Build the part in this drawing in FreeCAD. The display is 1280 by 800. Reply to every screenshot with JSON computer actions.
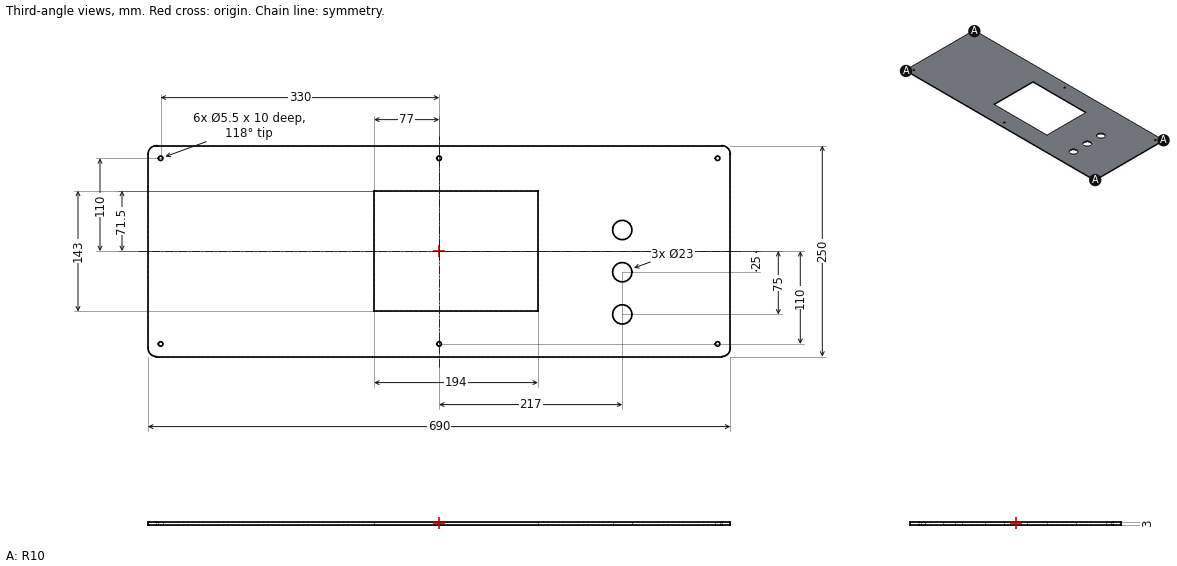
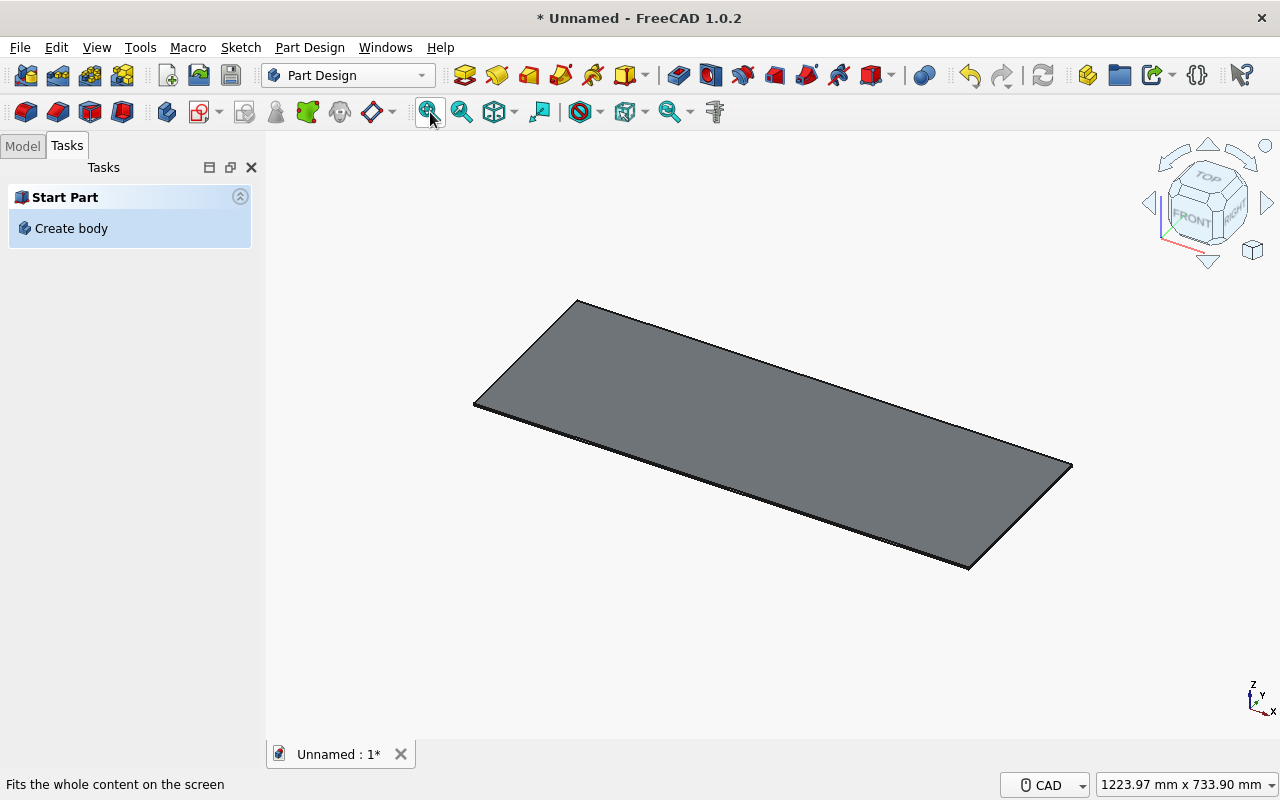
{"action": "left_click", "coordinate": [914, 480]}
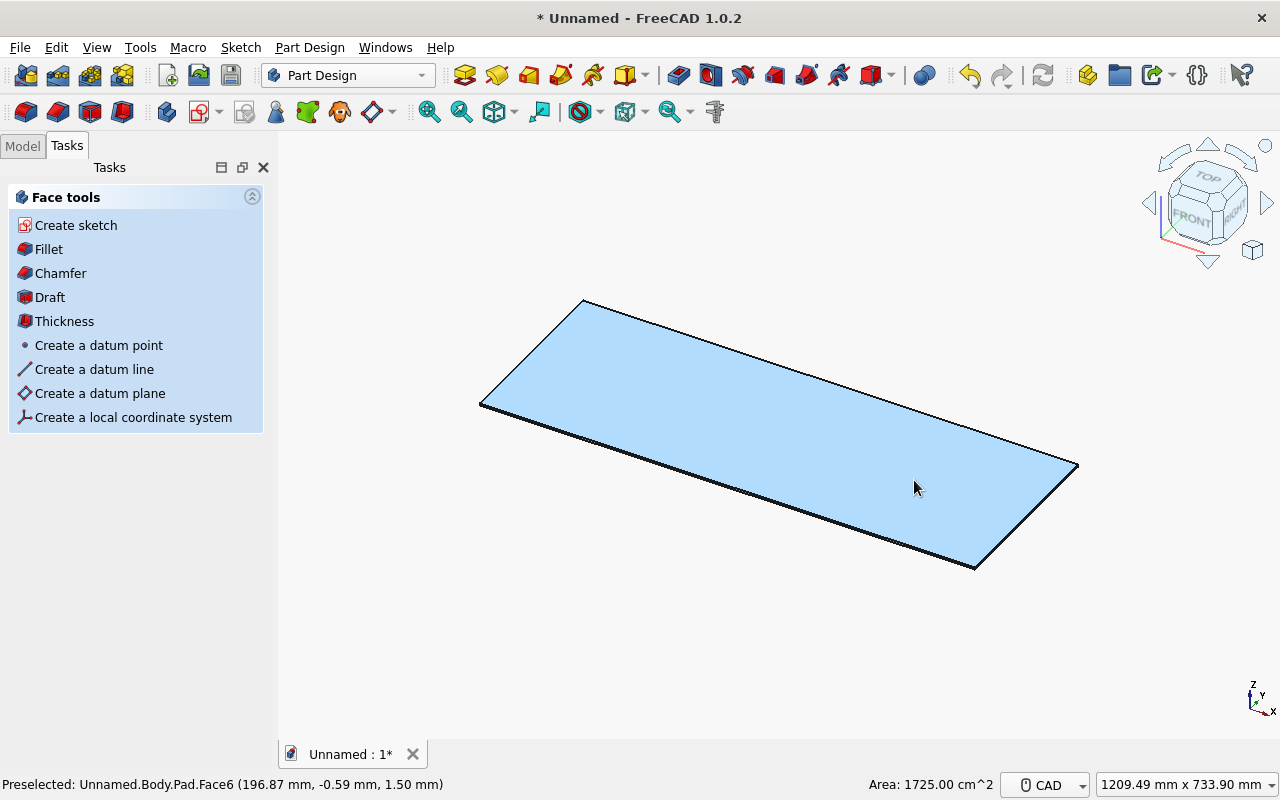
{"action": "left_click", "coordinate": [200, 112]}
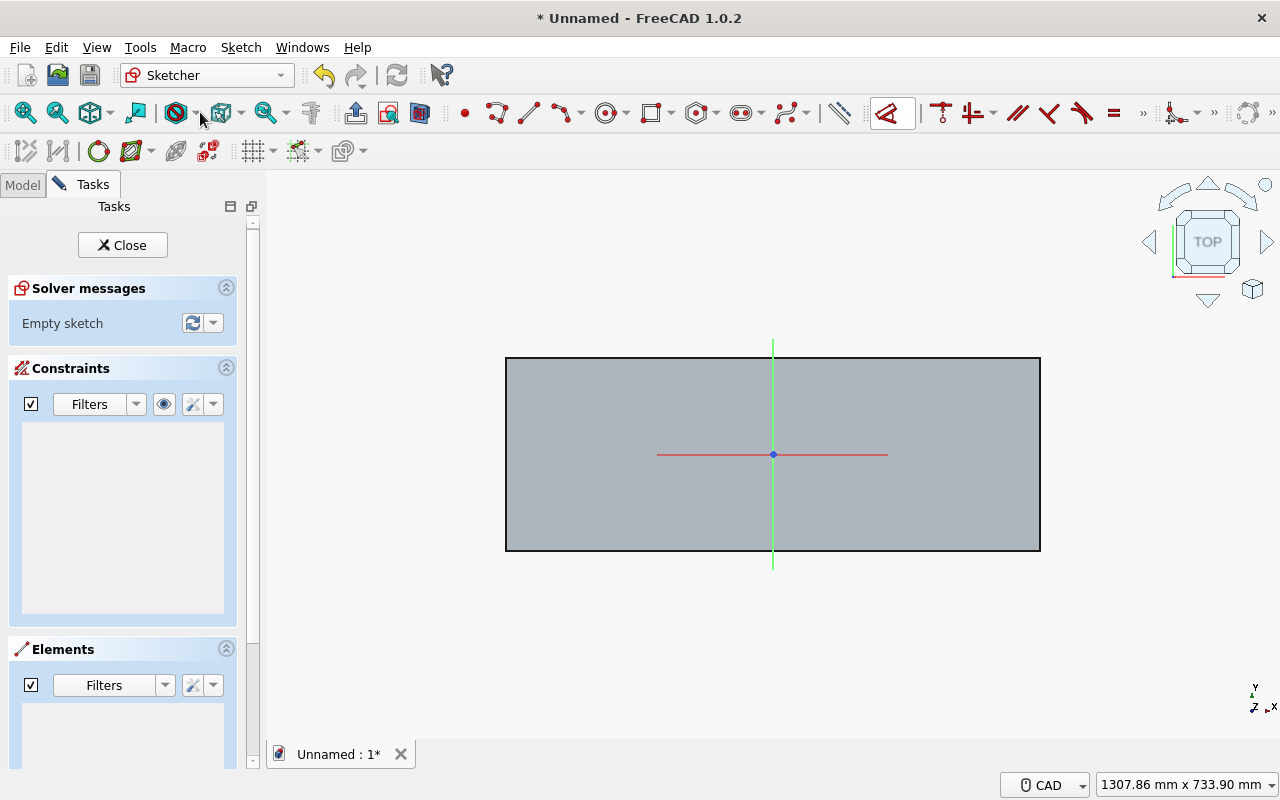
{"action": "scroll", "coordinate": [825, 455], "scroll_direction": "up", "scroll_amount": 6}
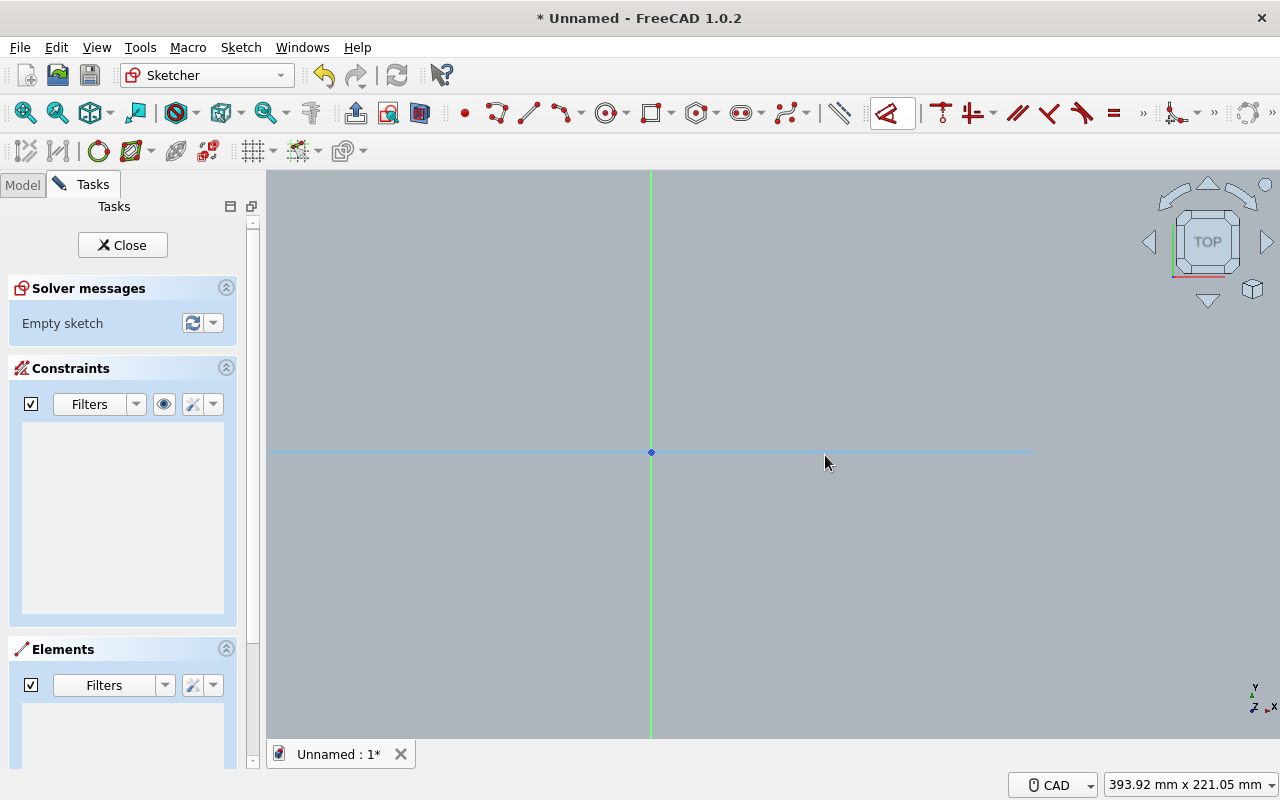
{"action": "left_click", "coordinate": [652, 114]}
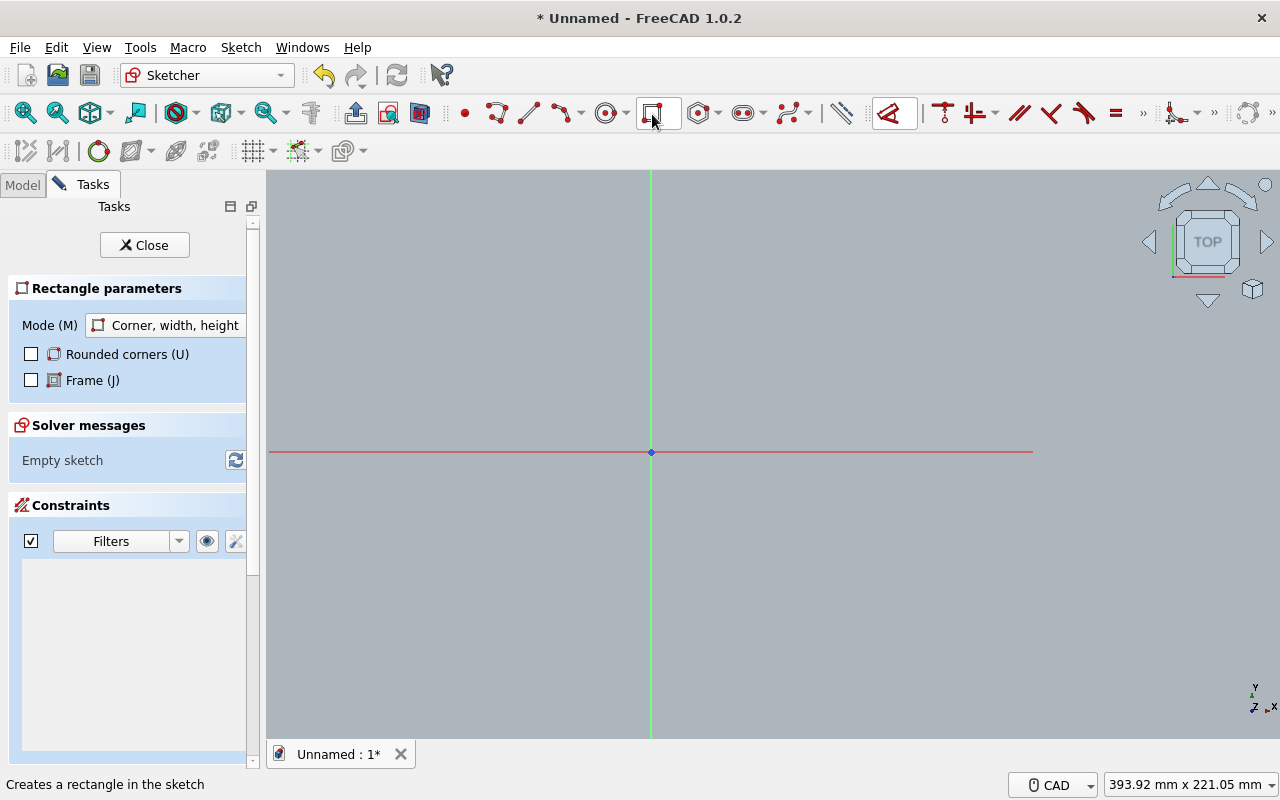
{"action": "left_click", "coordinate": [453, 268]}
{"action": "left_click", "coordinate": [952, 636]}
{"action": "key", "text": "Escape"}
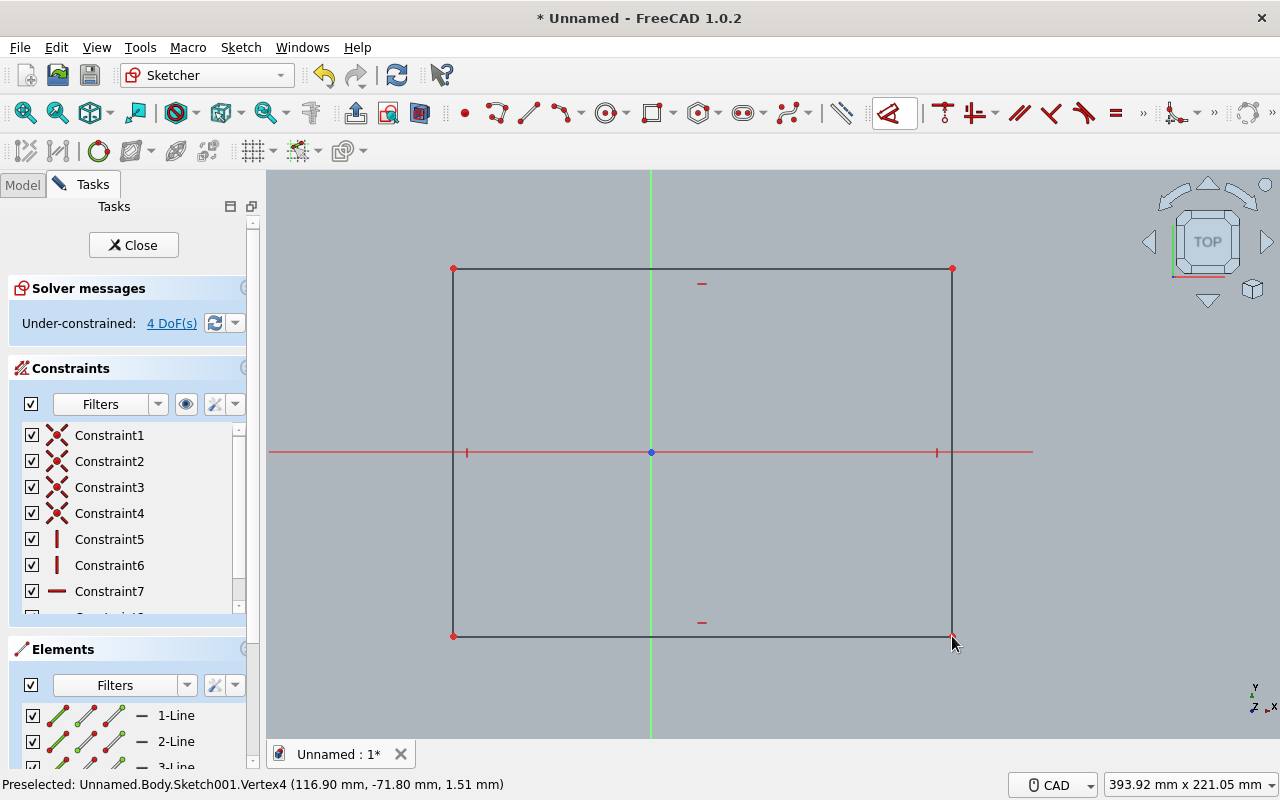
{"action": "left_click", "coordinate": [453, 379]}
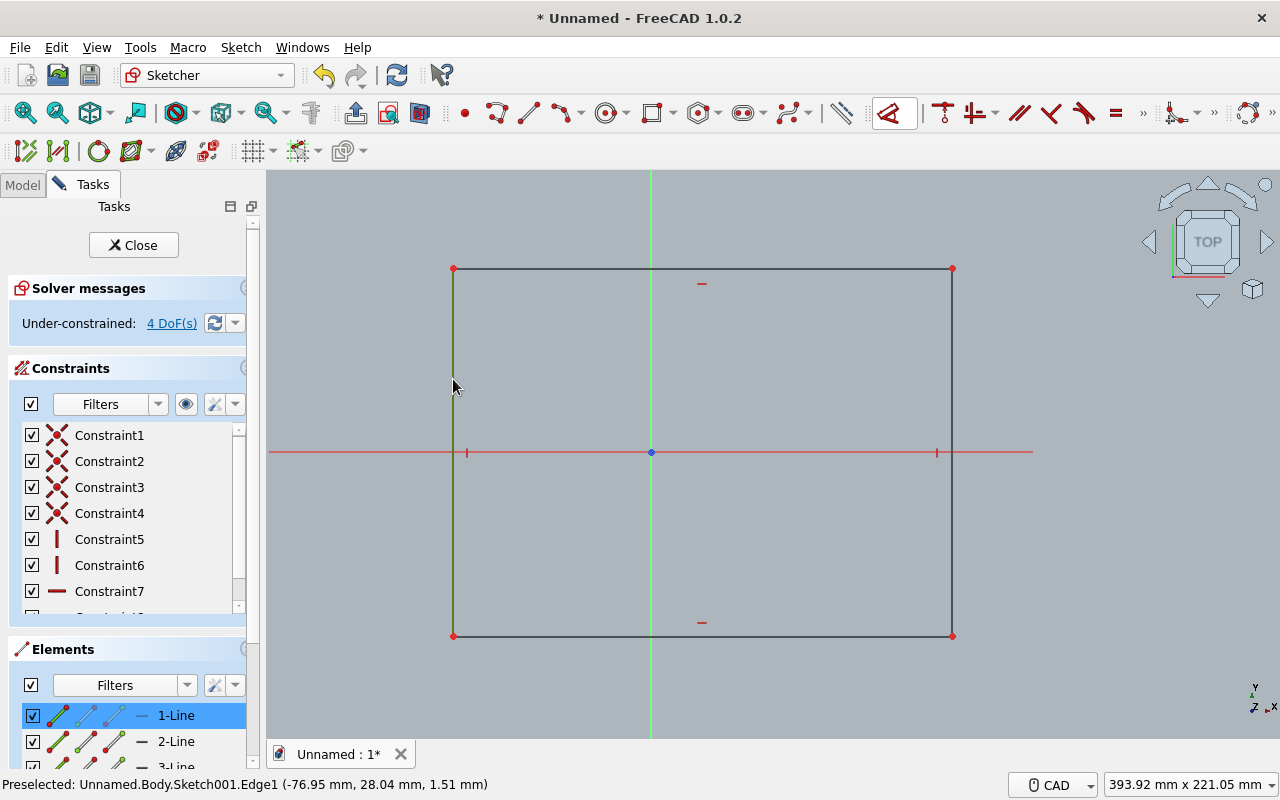
{"action": "left_click", "coordinate": [912, 114]}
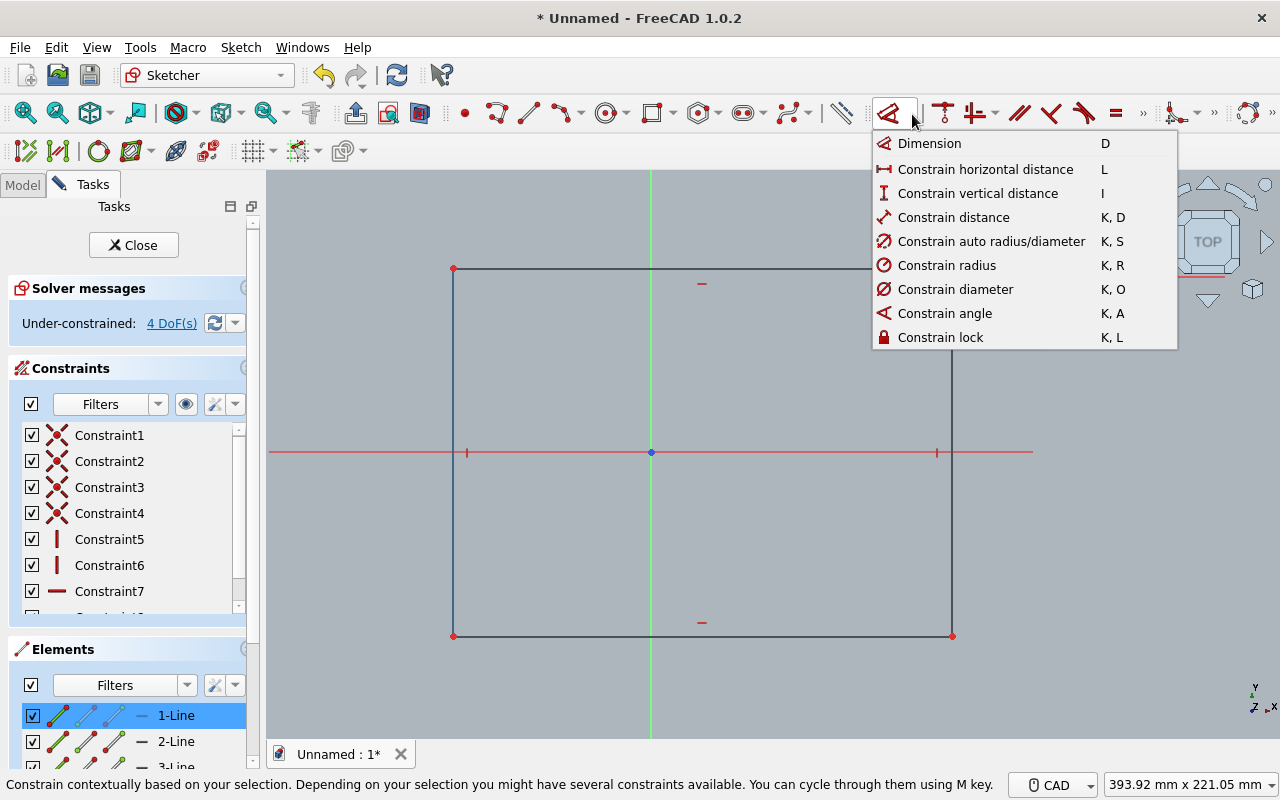
{"action": "left_click", "coordinate": [1025, 193]}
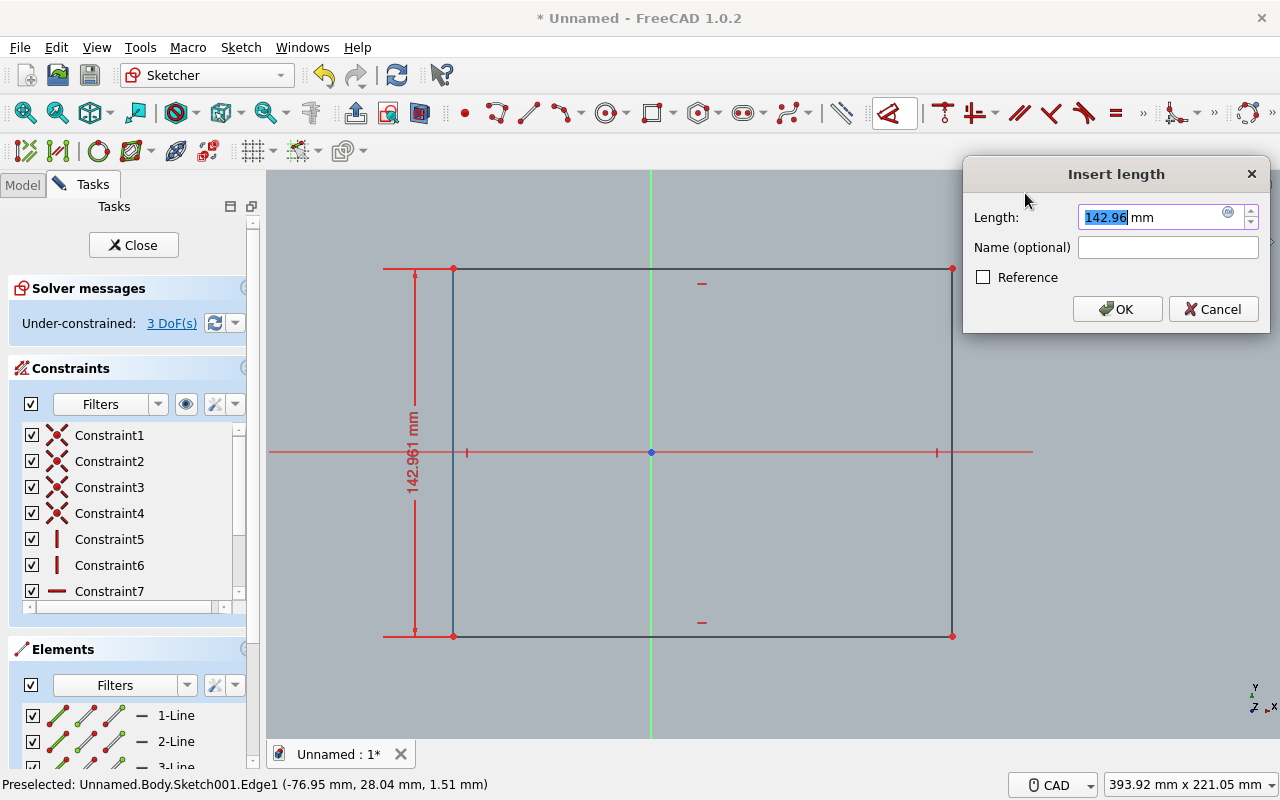
{"action": "type", "text": "143"}
{"action": "key", "text": "Return"}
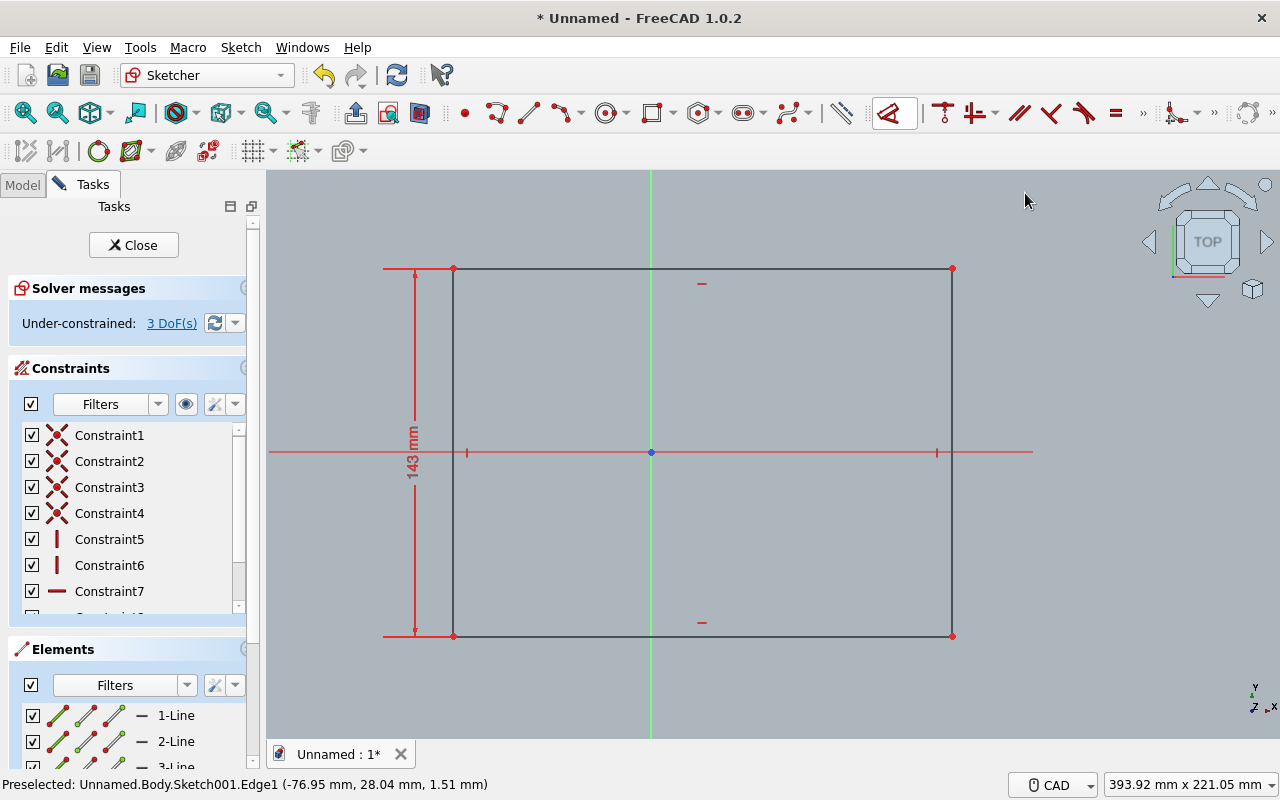
{"action": "left_click", "coordinate": [603, 637]}